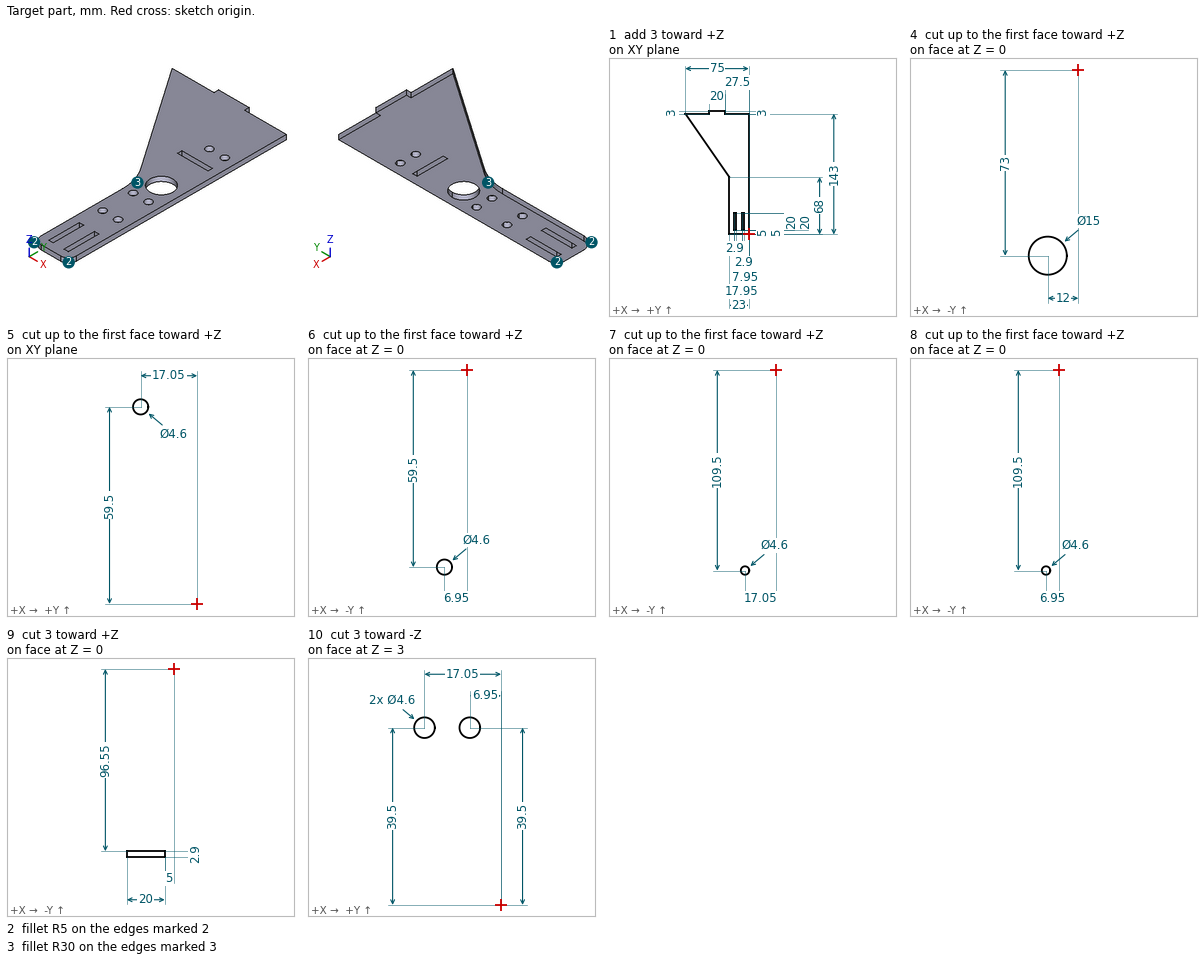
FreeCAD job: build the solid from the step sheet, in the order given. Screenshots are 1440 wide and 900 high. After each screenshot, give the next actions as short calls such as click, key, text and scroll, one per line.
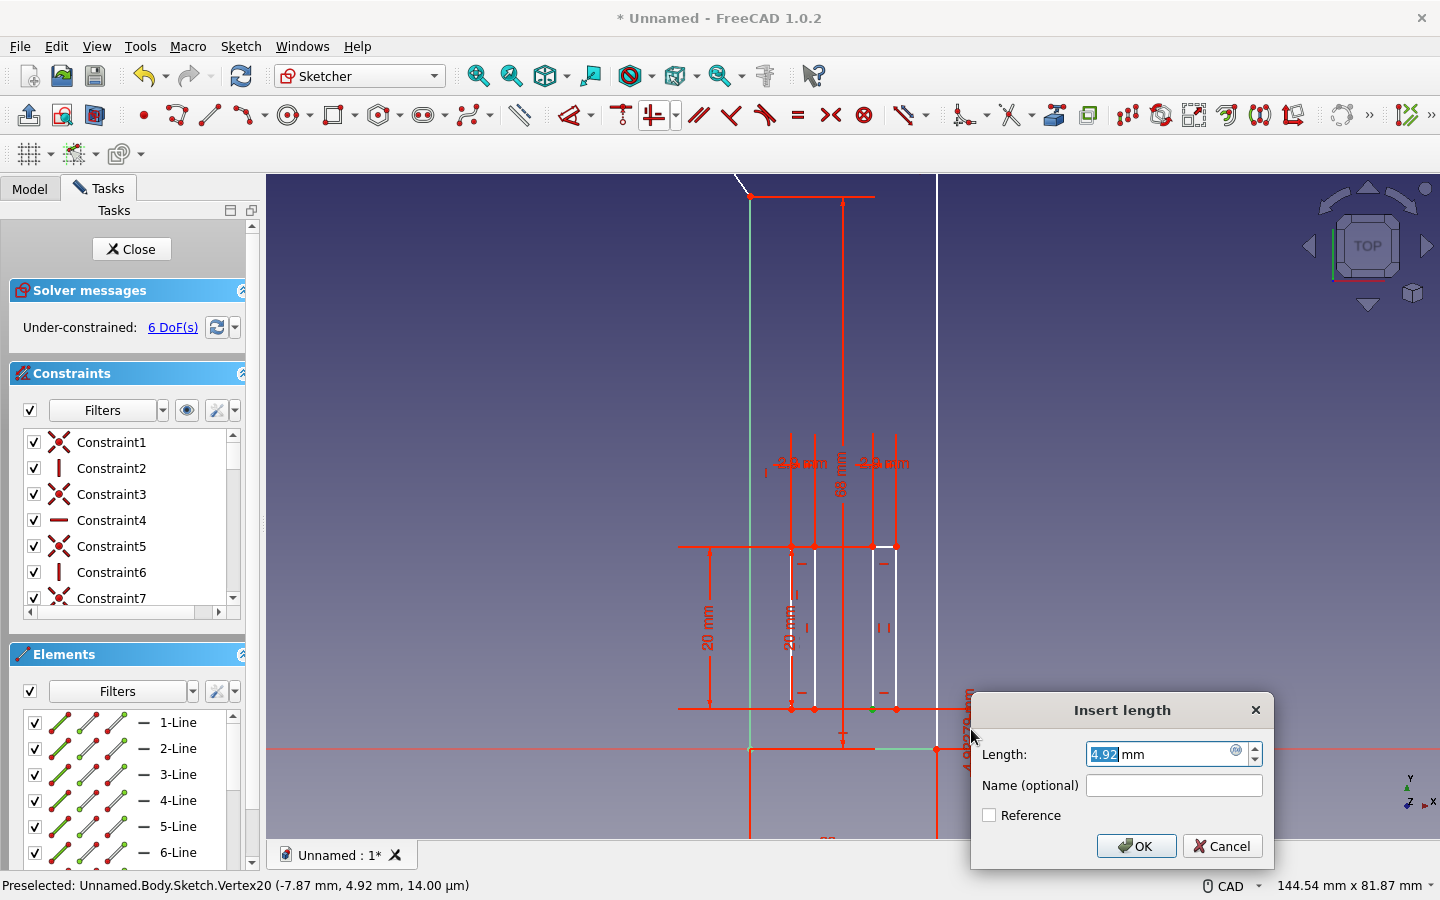
text(5)
key(Return)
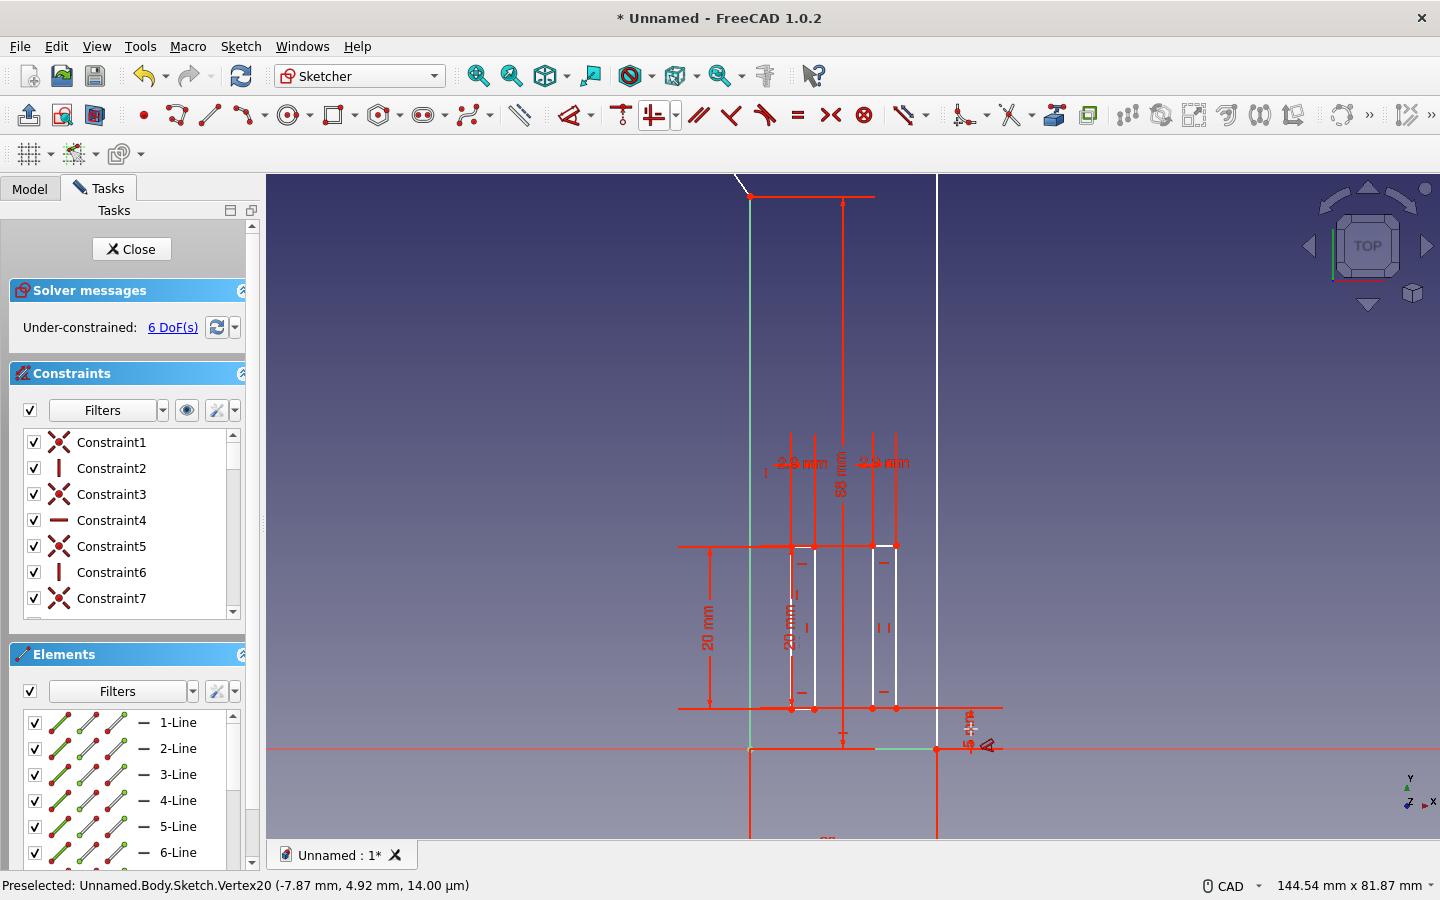
click(791, 709)
click(733, 729)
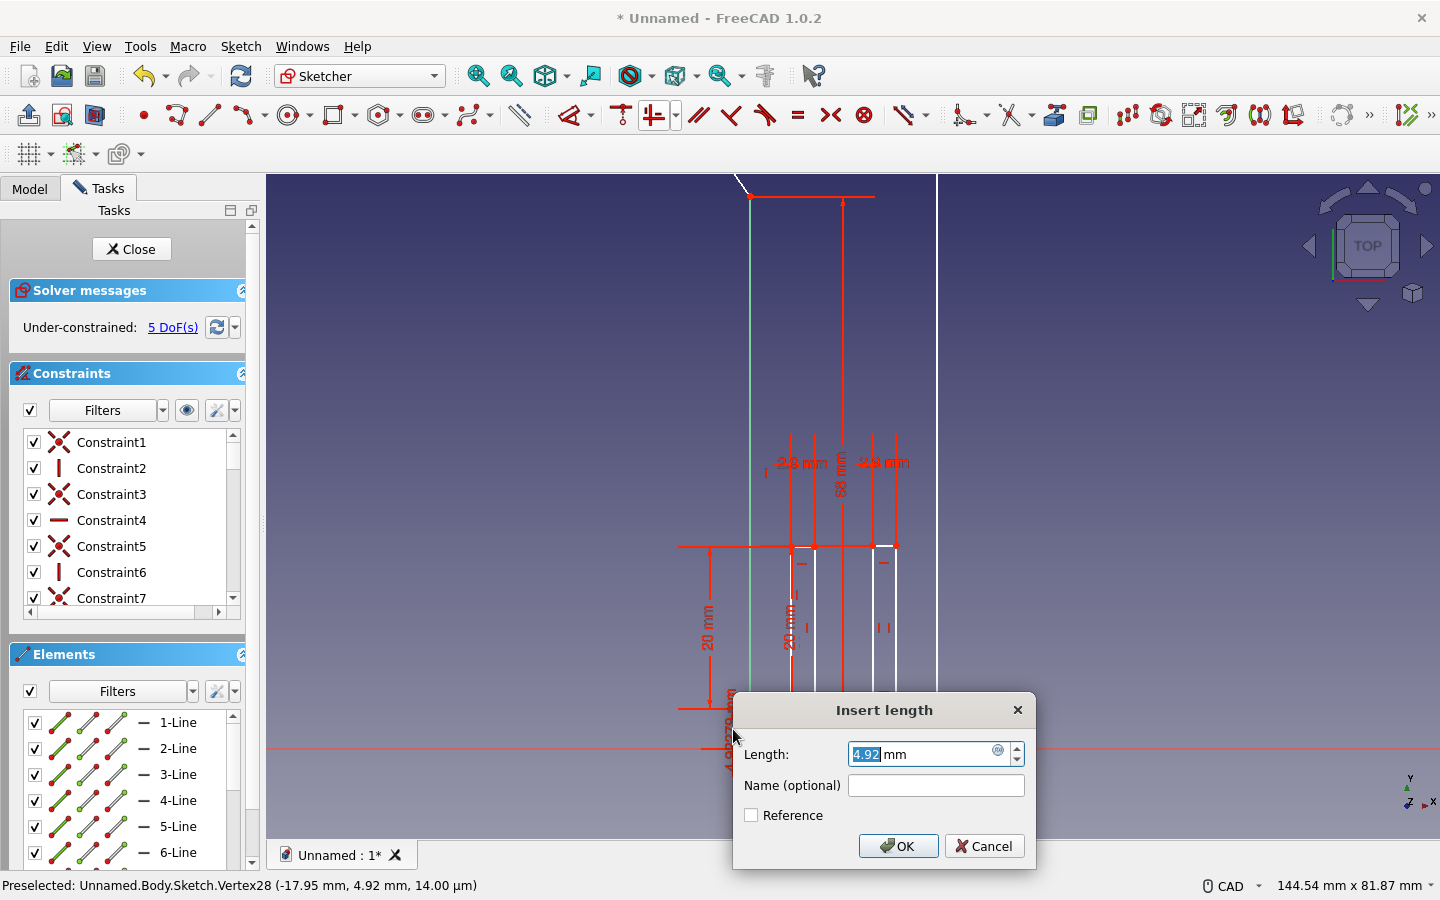
text(5)
key(Return)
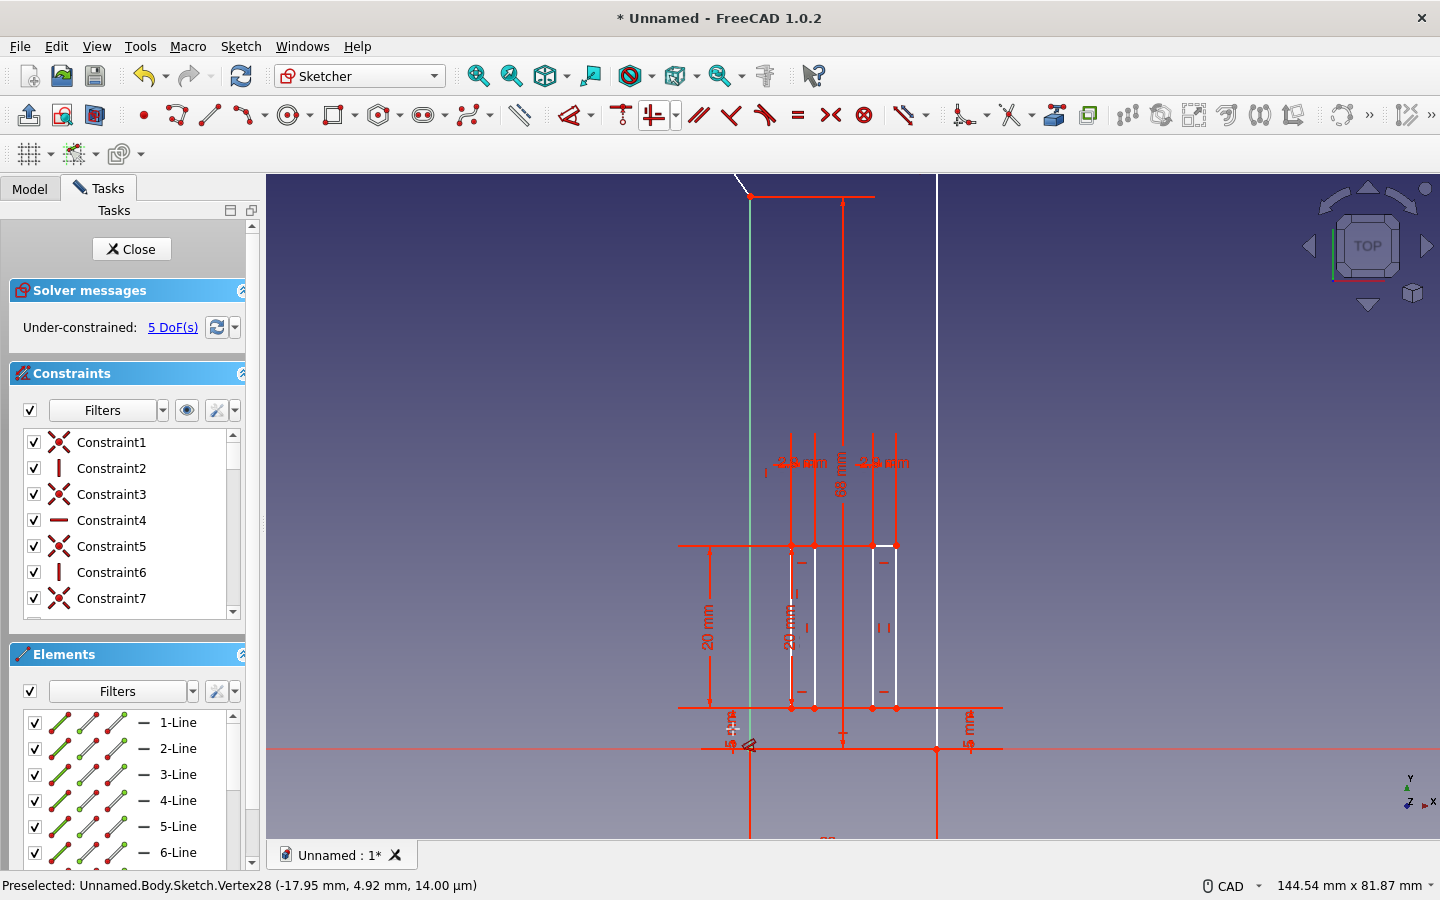
click(937, 401)
click(971, 476)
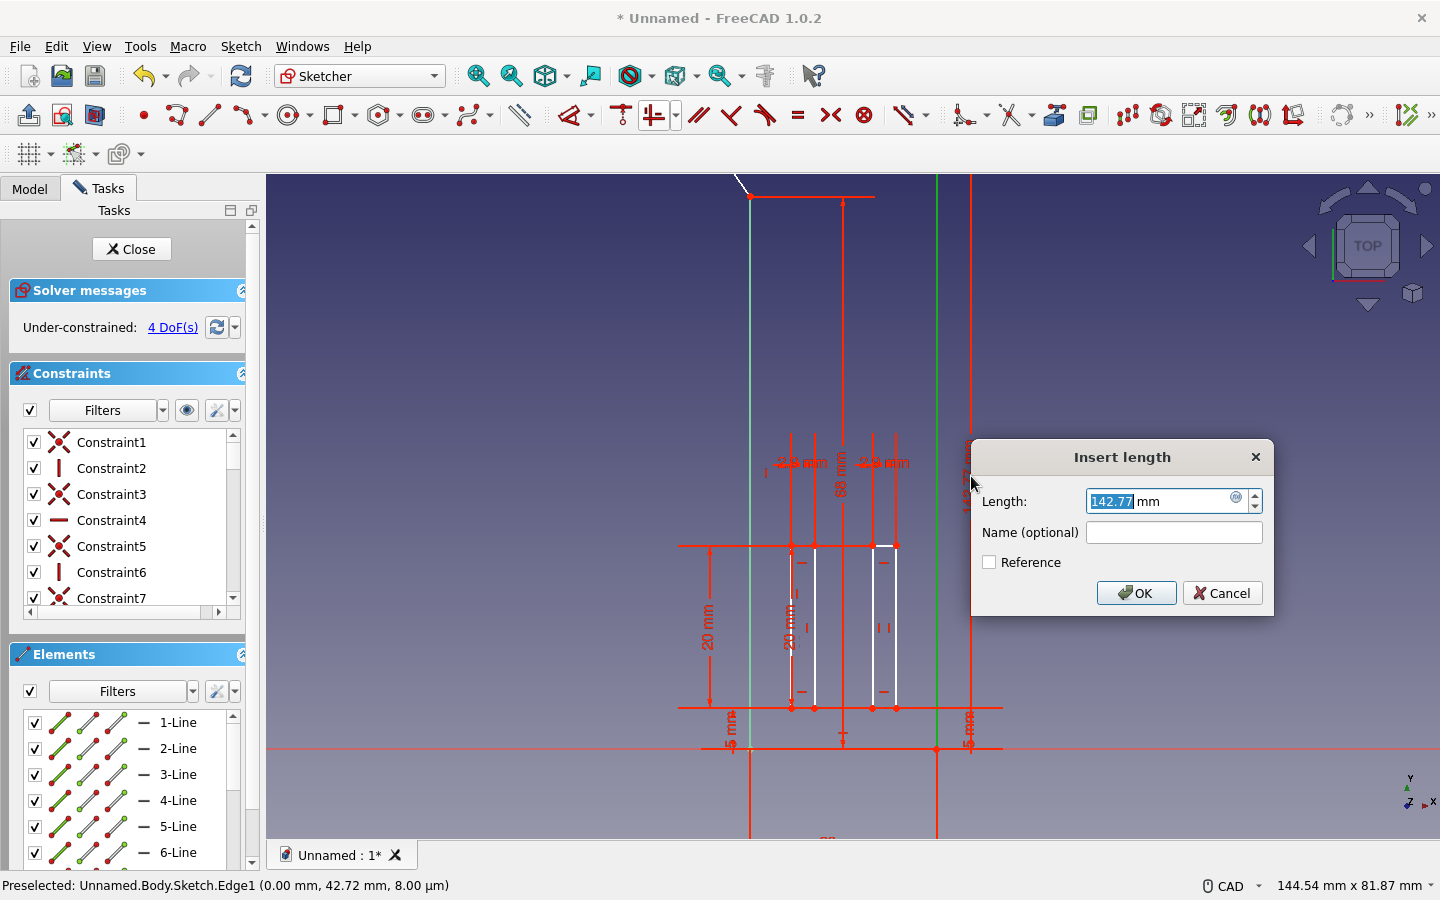
text(143)
key(Return)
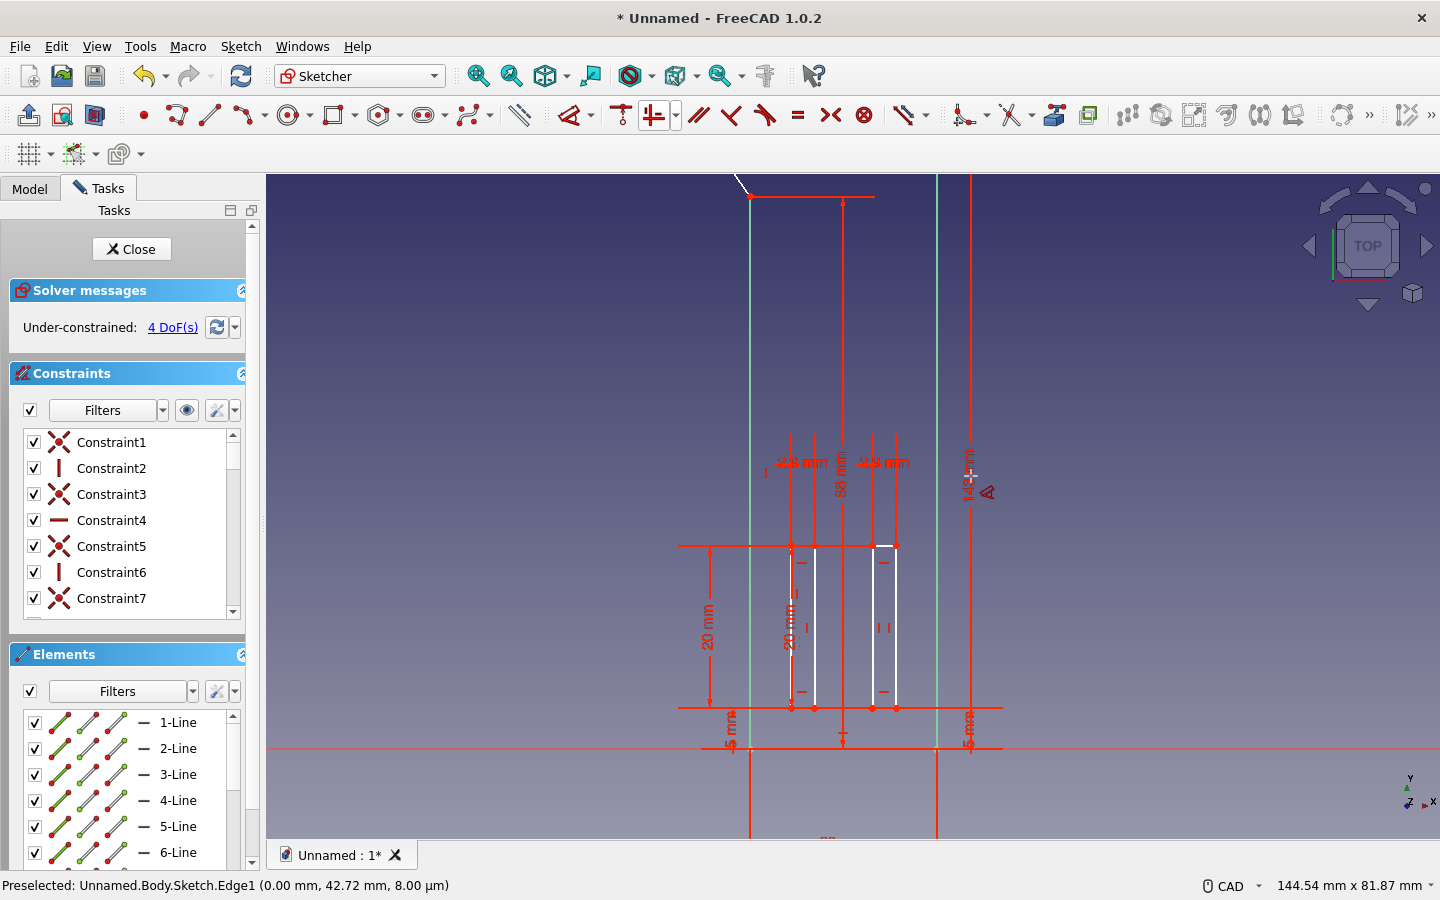
scroll(873, 710, down, 5)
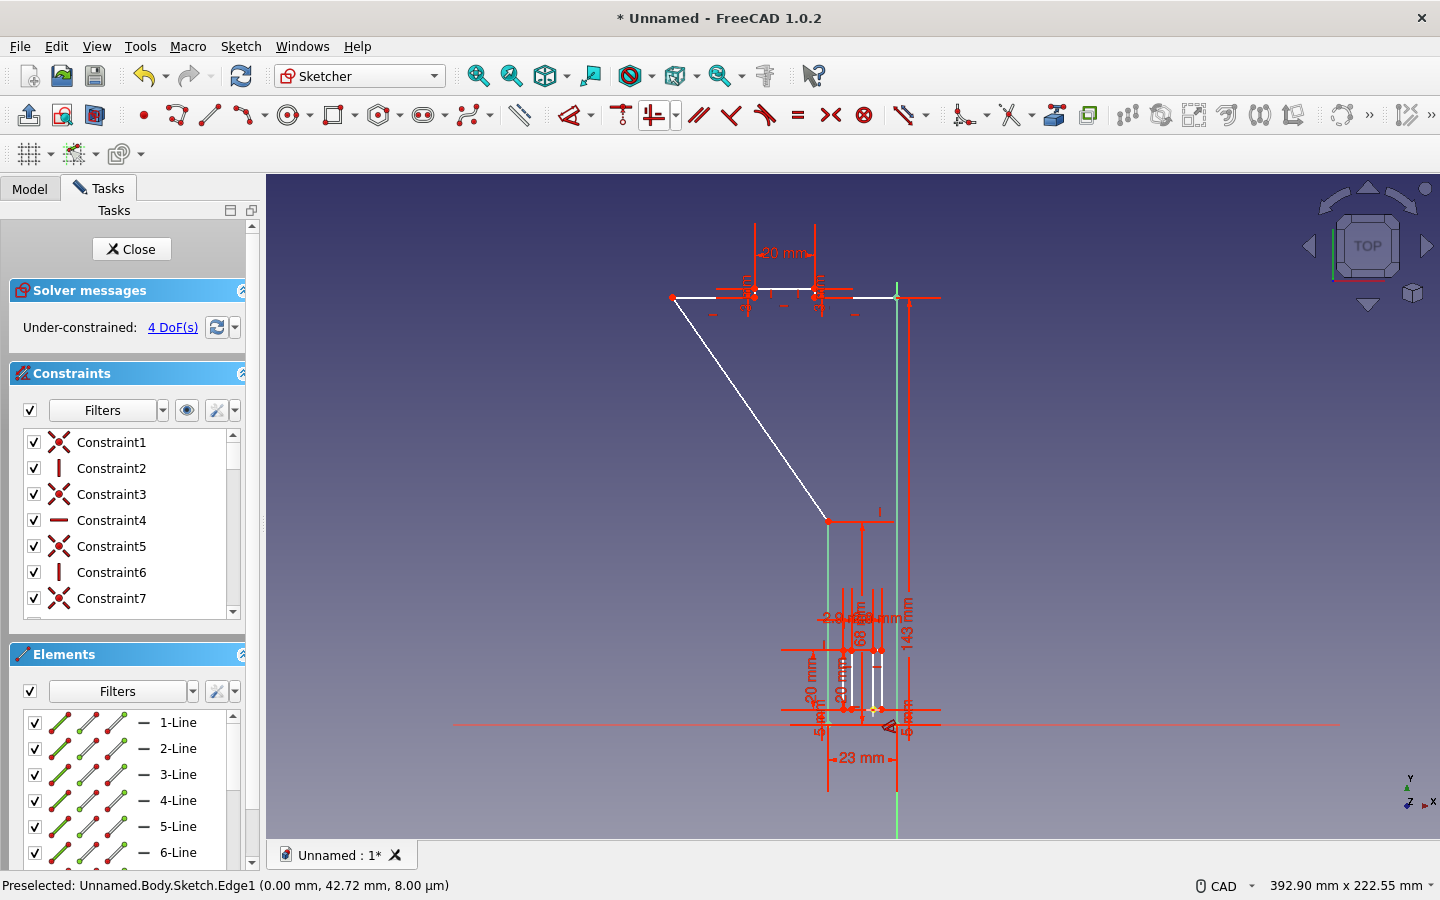
click(673, 298)
click(785, 759)